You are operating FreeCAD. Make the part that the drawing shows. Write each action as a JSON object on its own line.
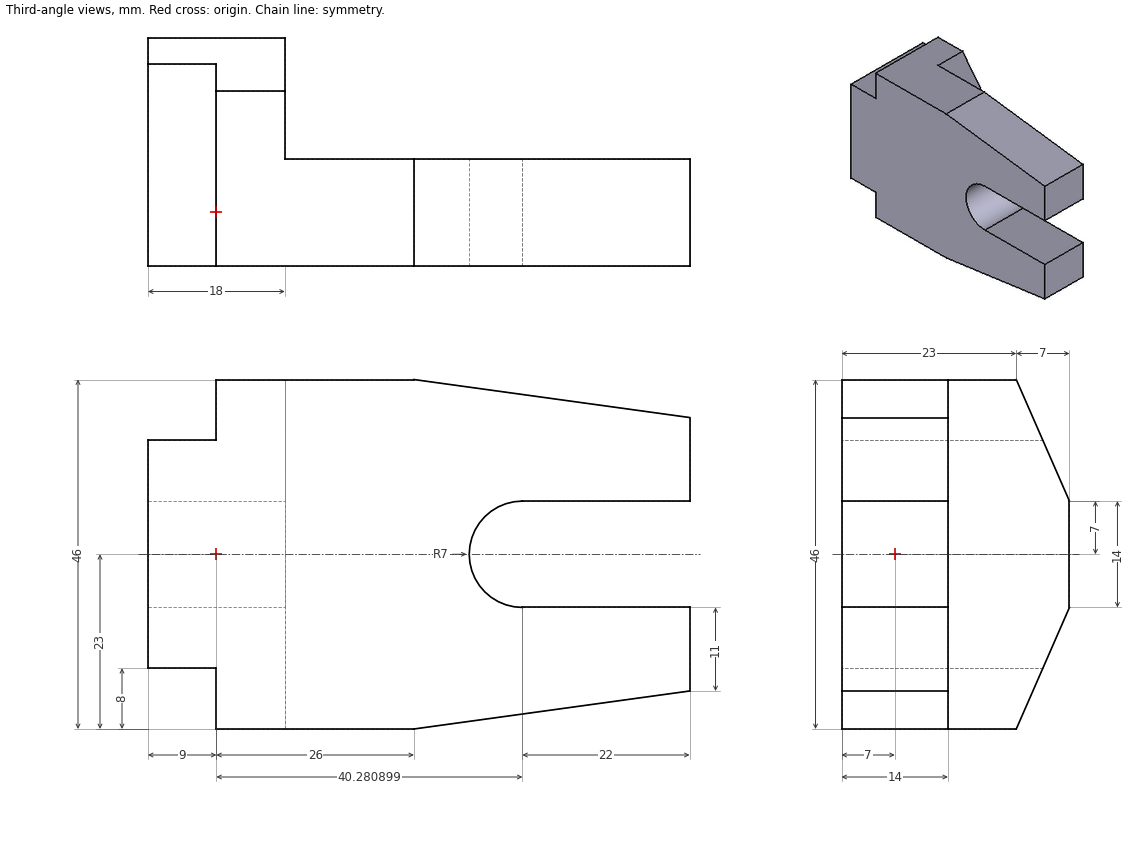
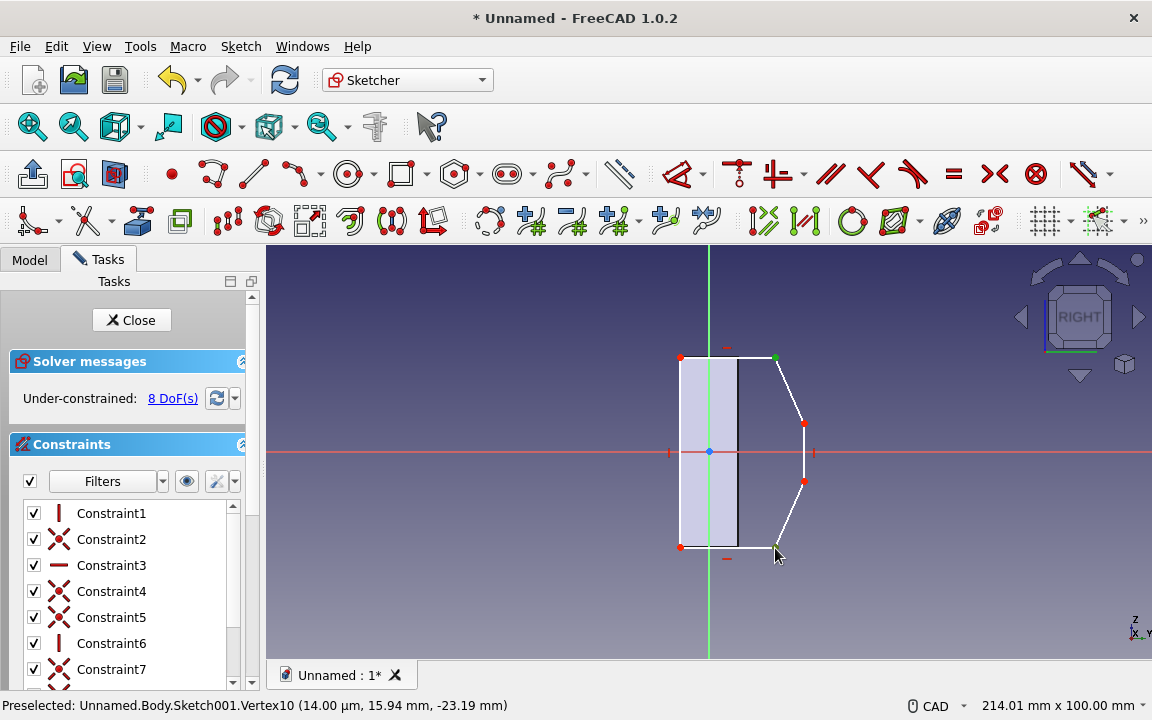
{"action": "left_click", "coordinate": [344, 452]}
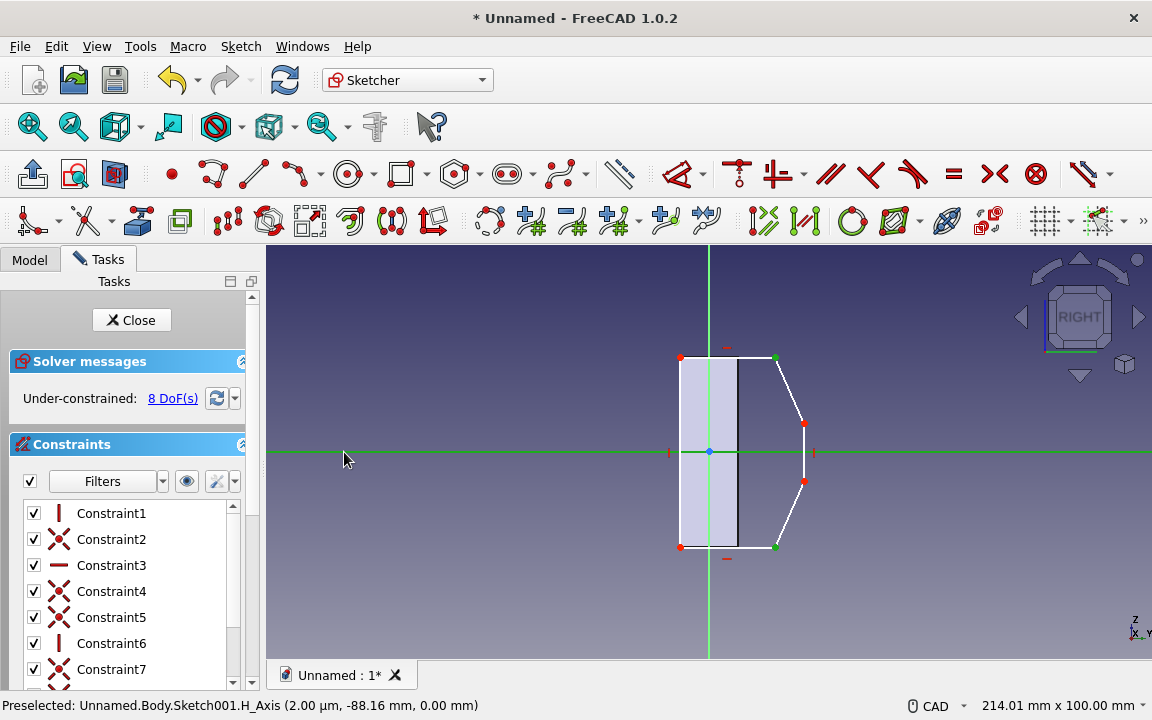
{"action": "left_click", "coordinate": [995, 174]}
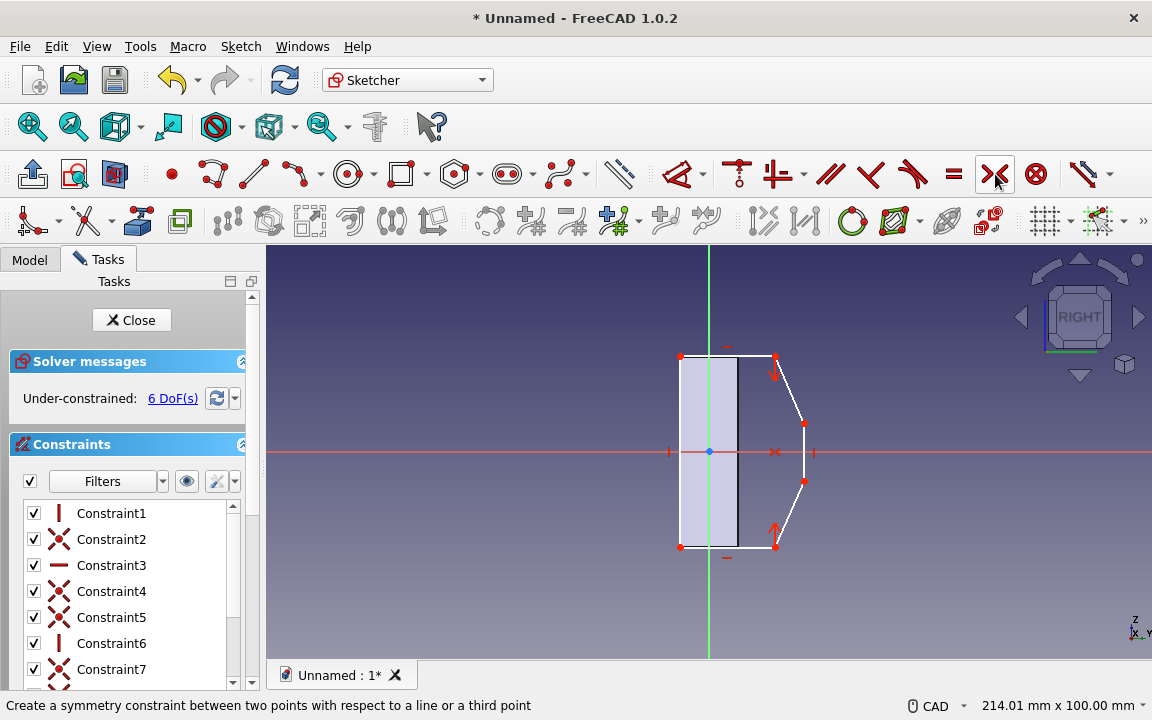
{"action": "left_click", "coordinate": [680, 490]}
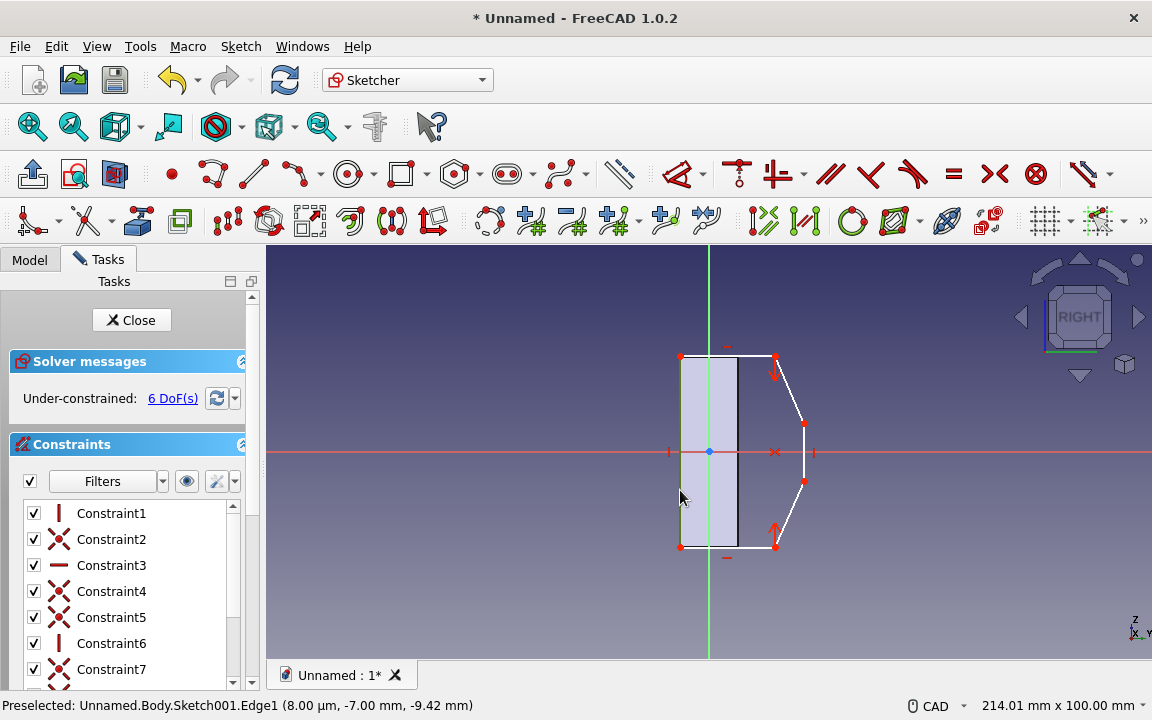
{"action": "left_click", "coordinate": [702, 174]}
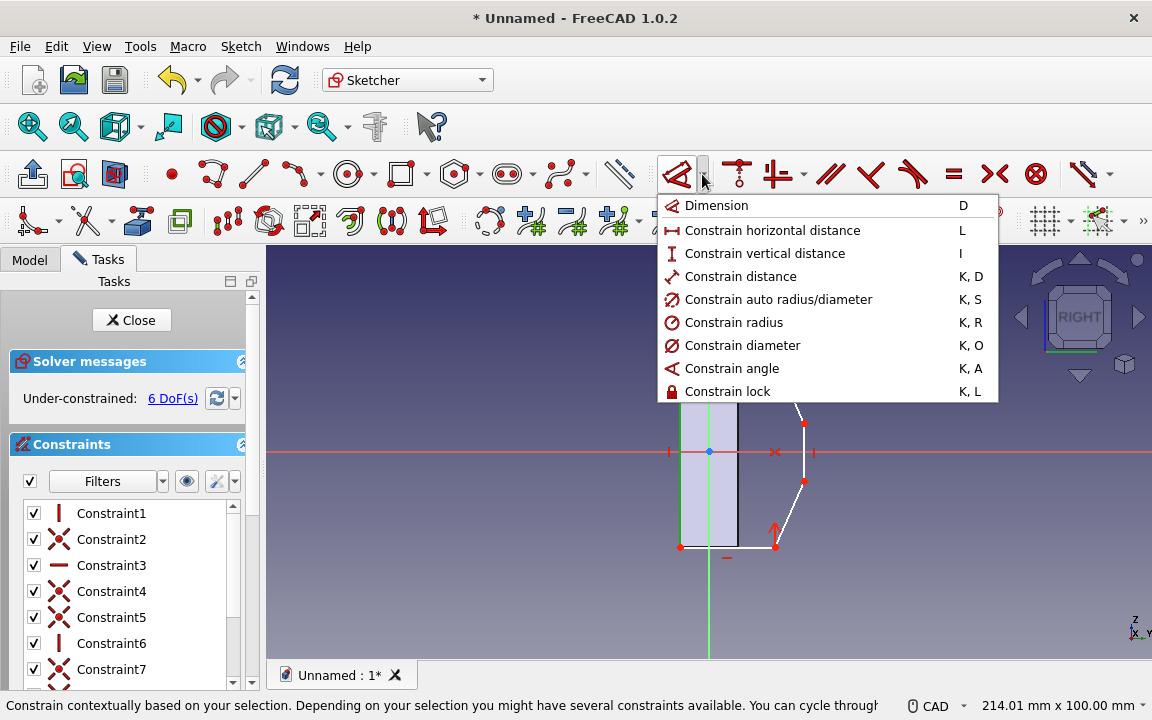
{"action": "left_click", "coordinate": [828, 254]}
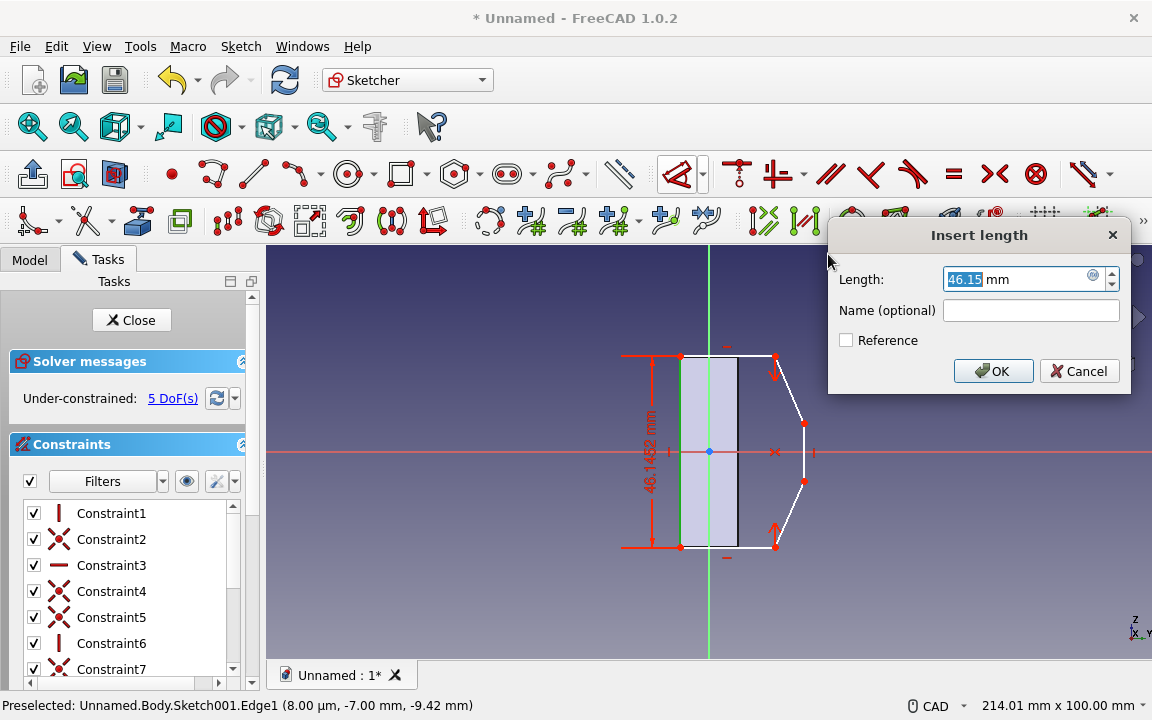
{"action": "type", "text": "46"}
{"action": "key", "text": "Return"}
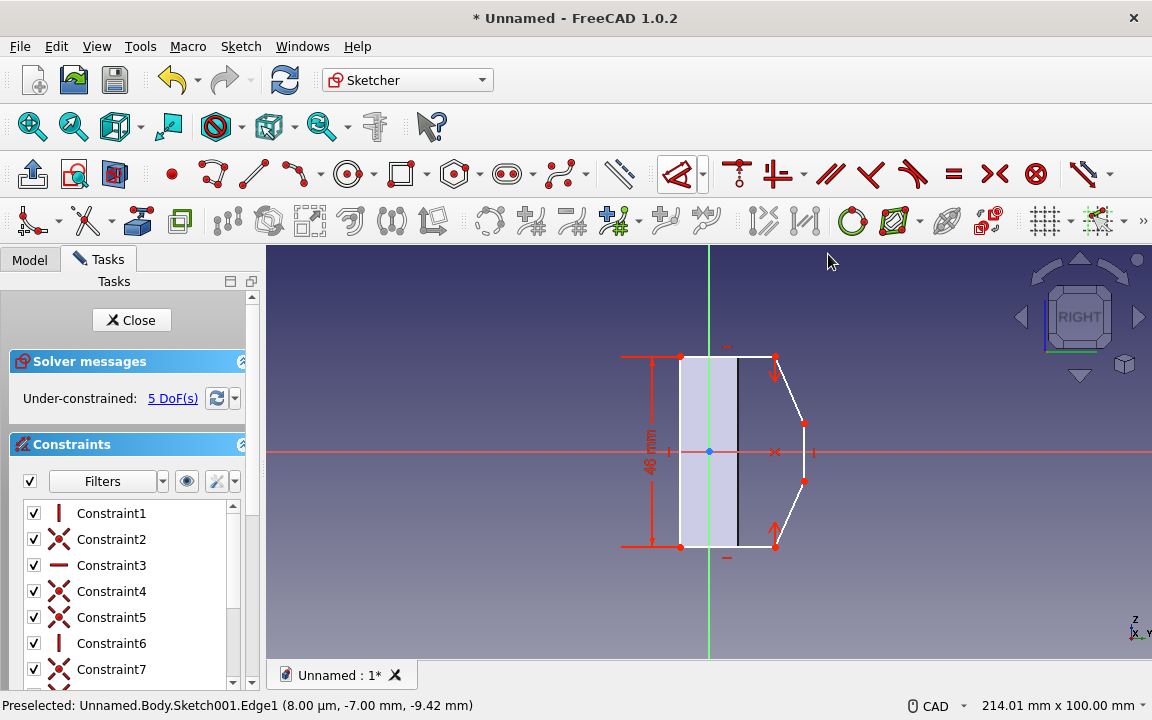
{"action": "left_click", "coordinate": [708, 357]}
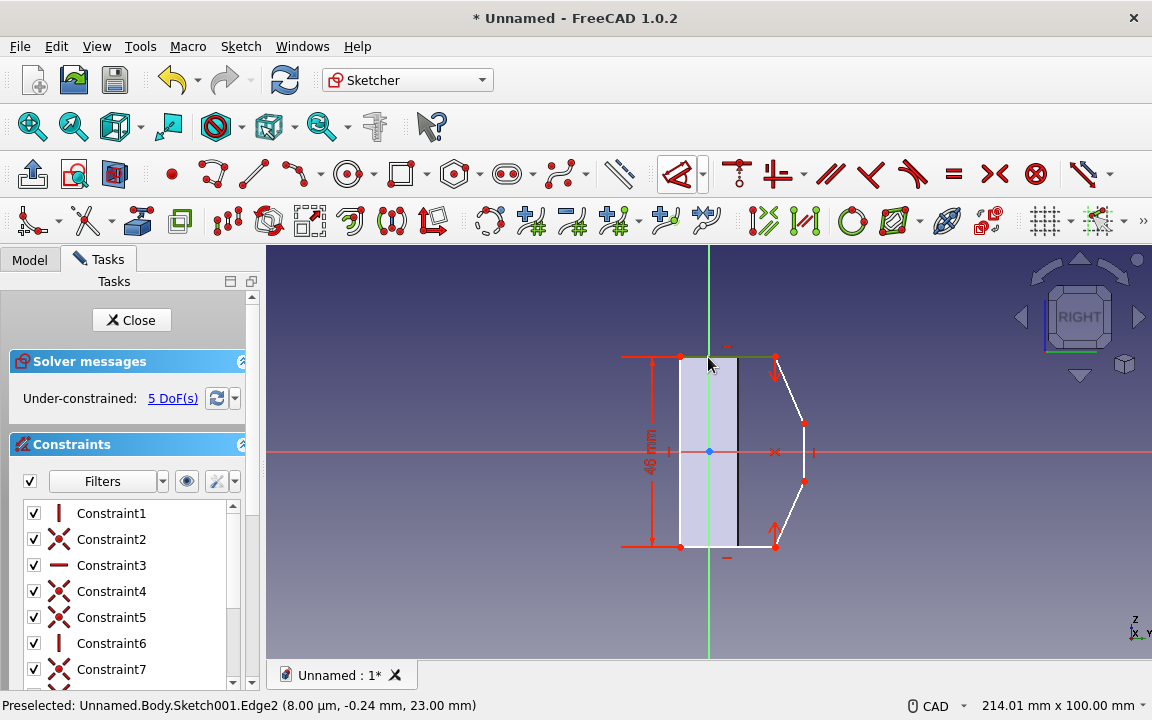
{"action": "key", "text": "l"}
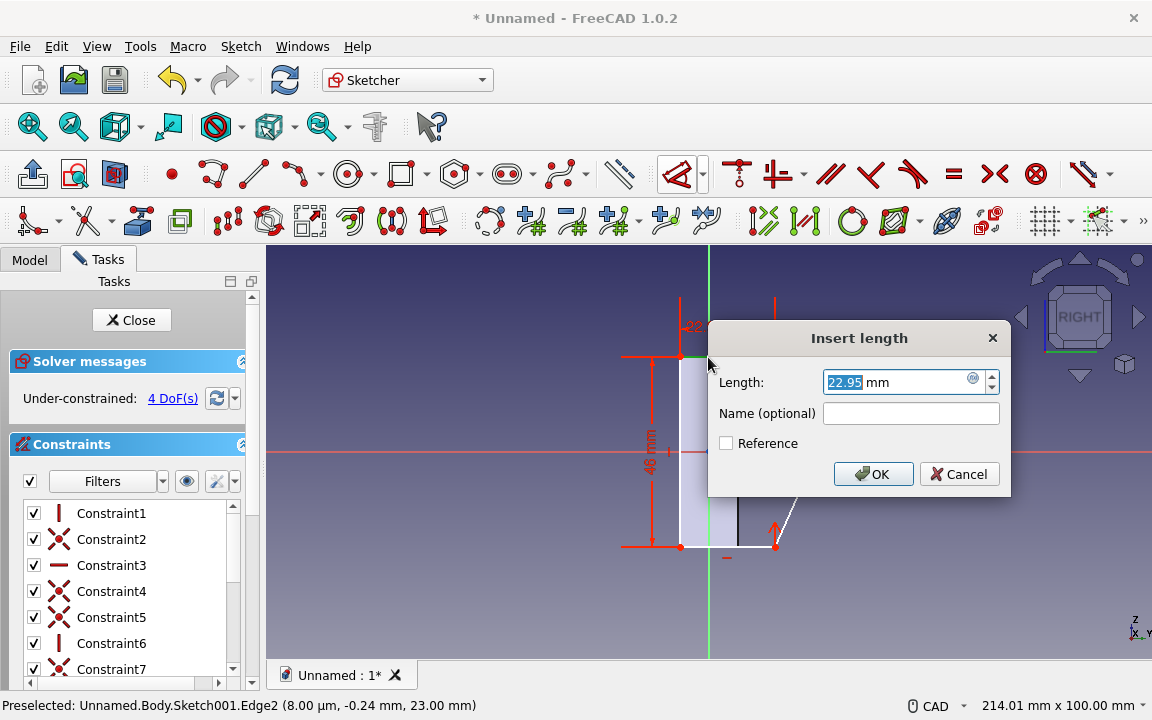
{"action": "type", "text": "23"}
{"action": "key", "text": "Return"}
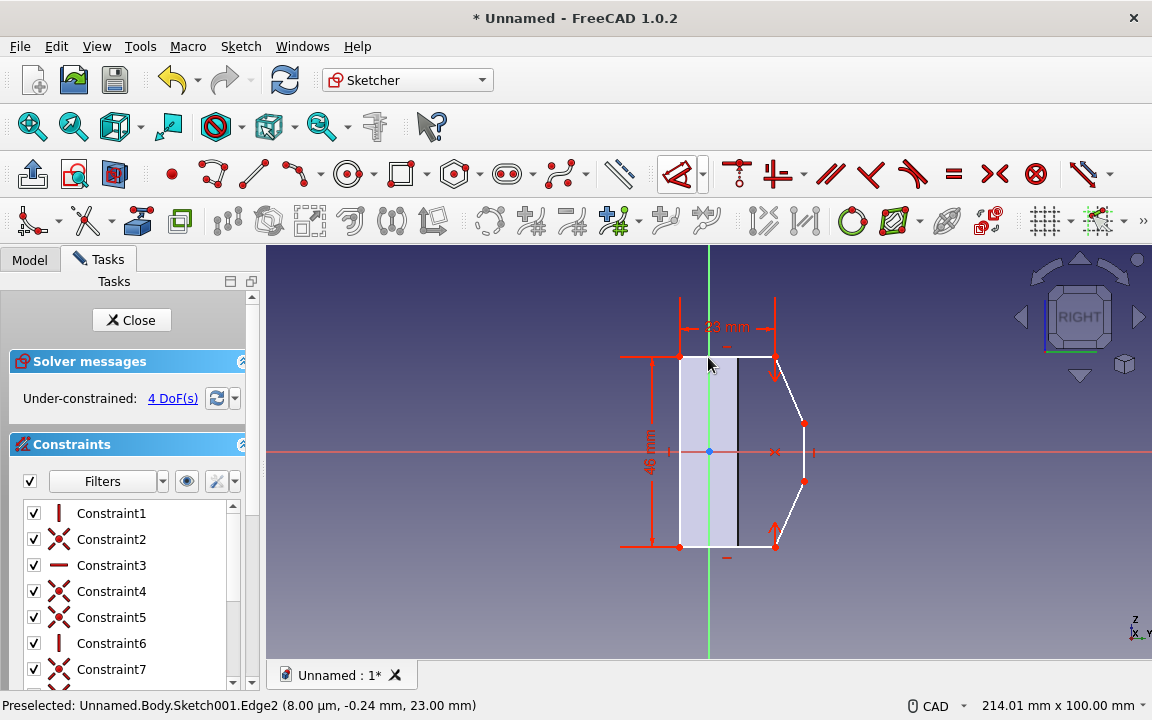
{"action": "scroll", "coordinate": [804, 441], "scroll_direction": "up", "scroll_amount": 2}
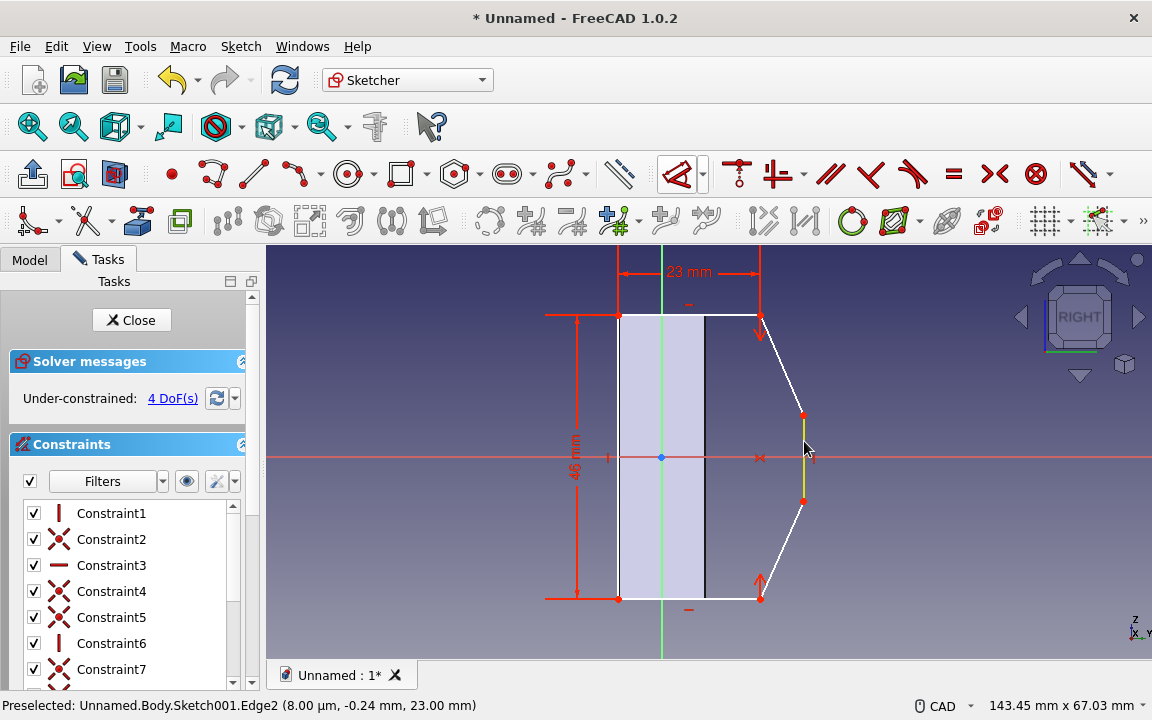
{"action": "left_click", "coordinate": [804, 441]}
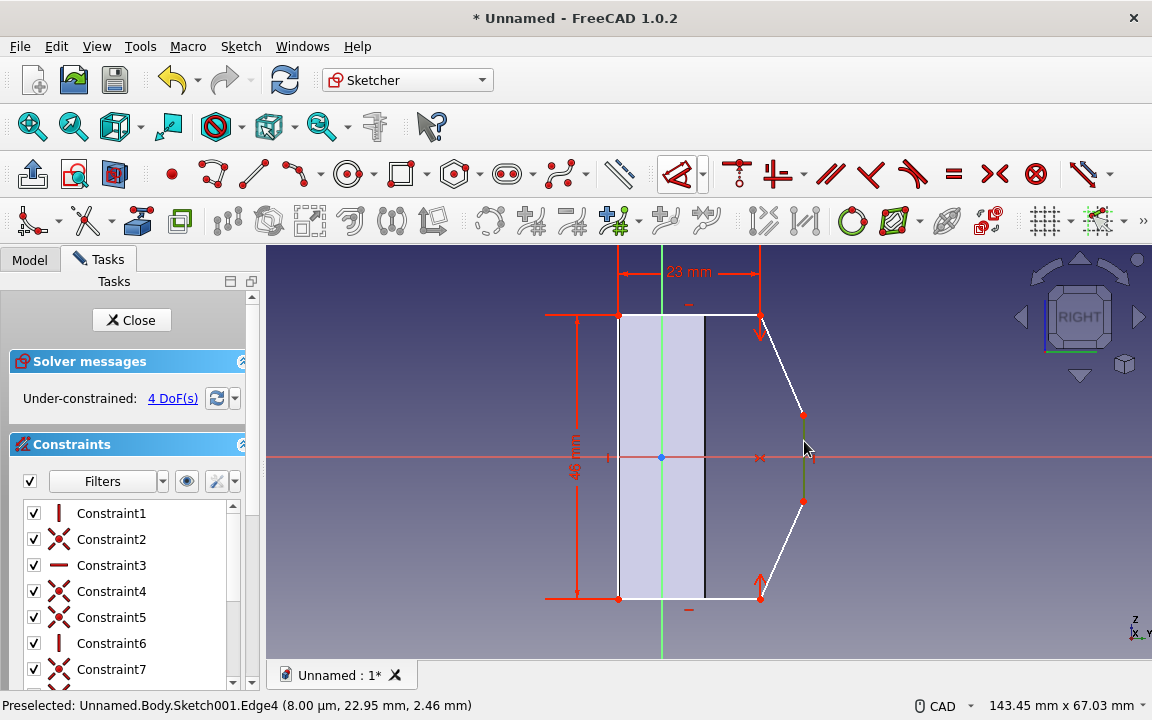
{"action": "key", "text": "i"}